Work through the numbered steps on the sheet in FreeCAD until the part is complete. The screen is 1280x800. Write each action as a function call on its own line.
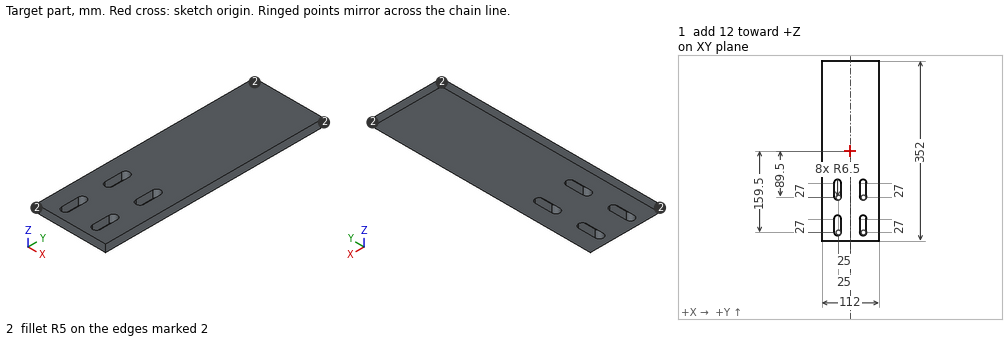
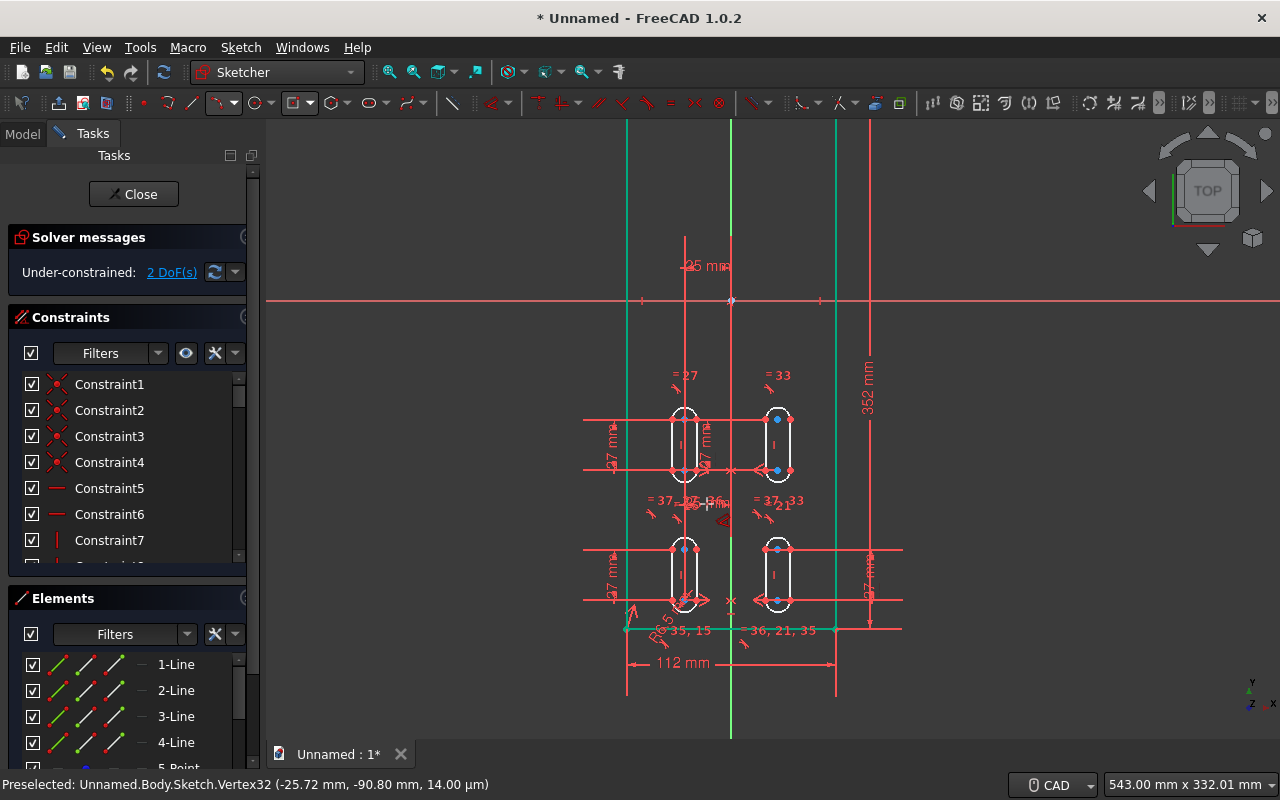
click(672, 470)
click(765, 385)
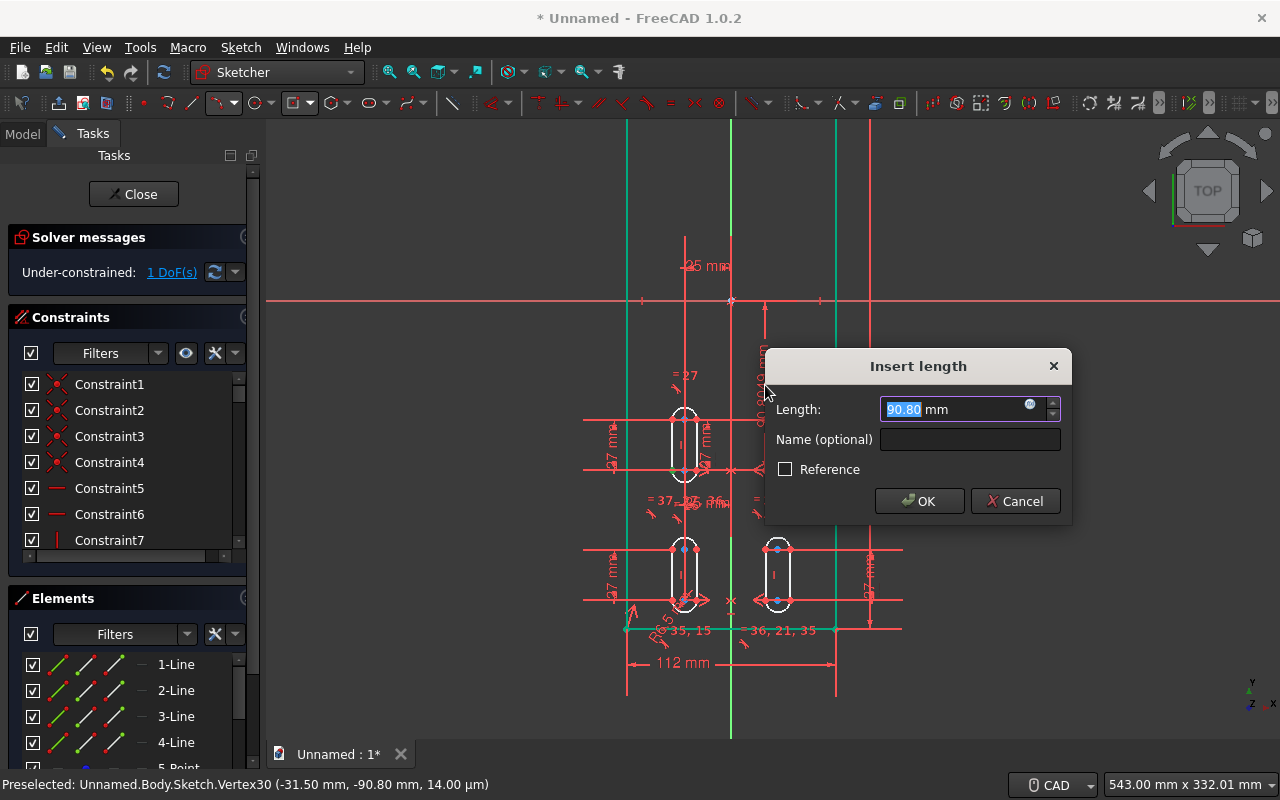
text(89.5)
key(Return)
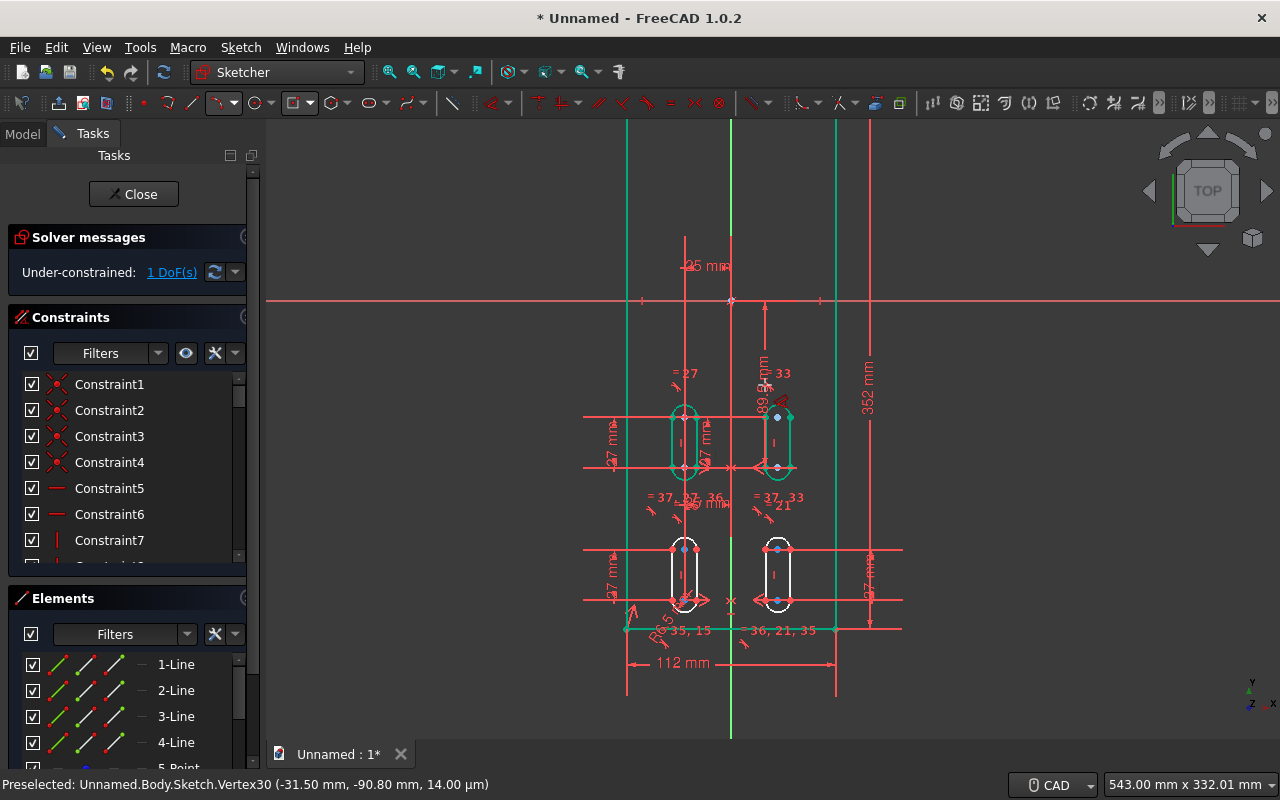
click(672, 600)
click(765, 346)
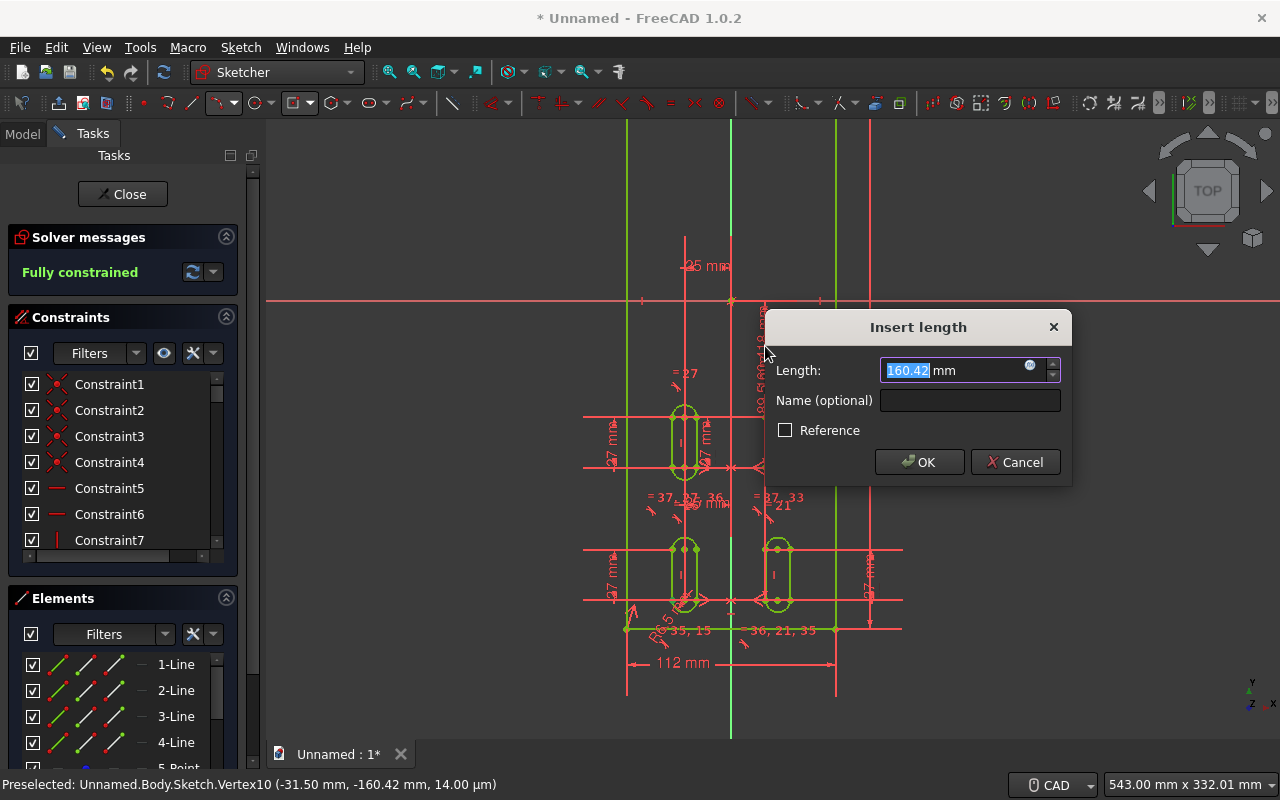
text(159.5)
key(Return)
key(Escape)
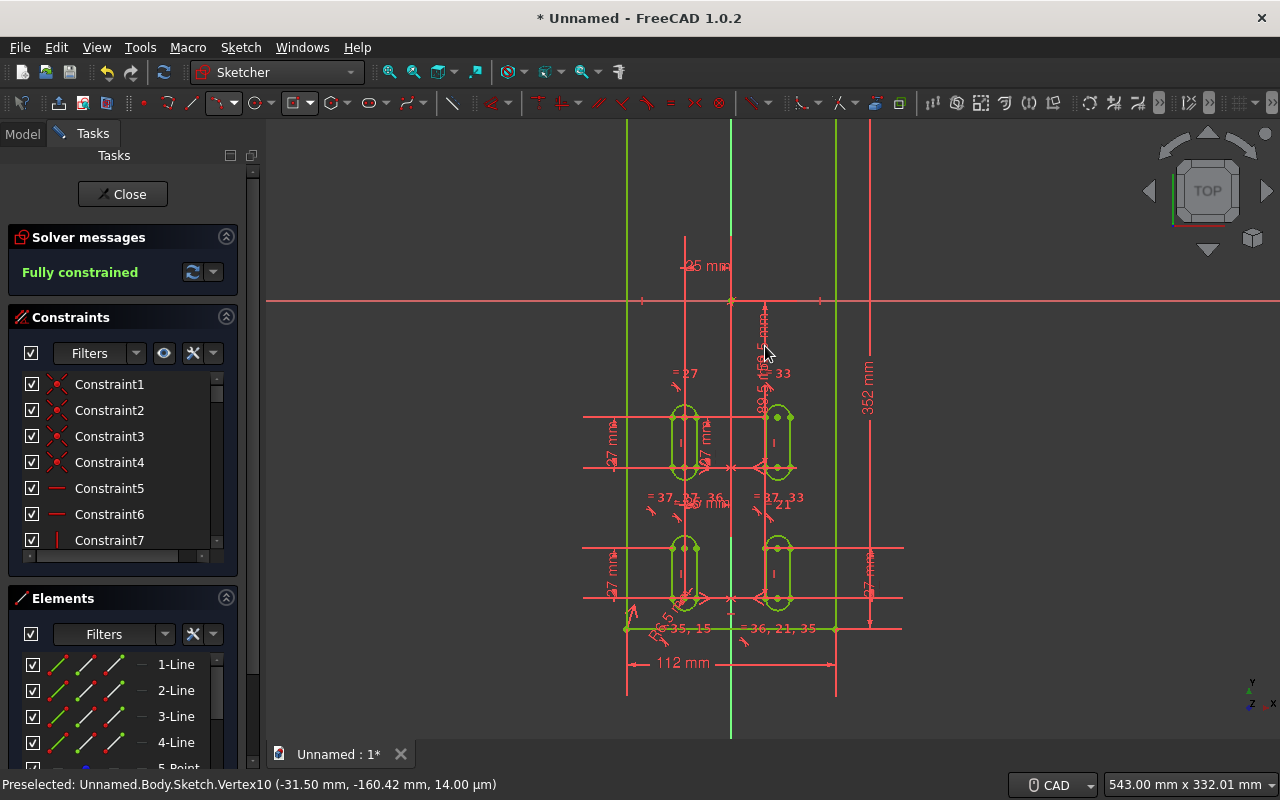
click(123, 194)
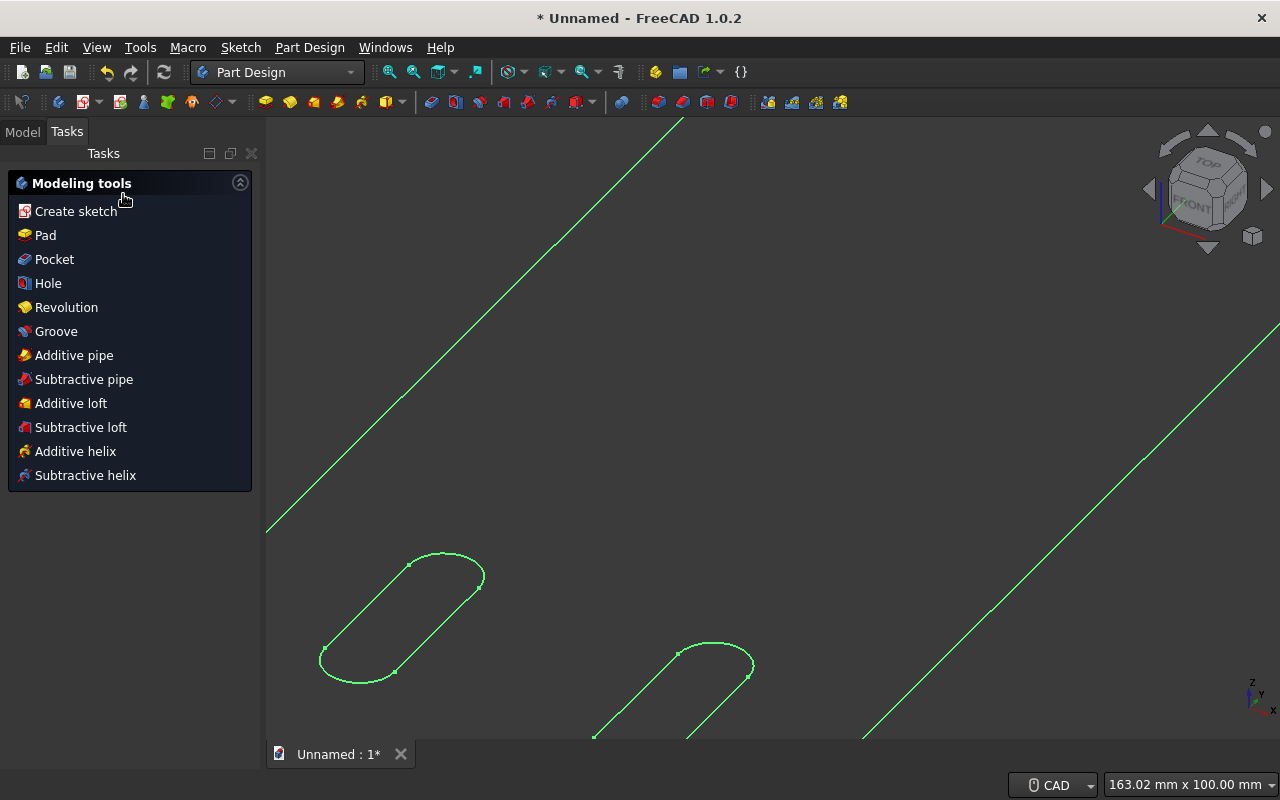
click(266, 102)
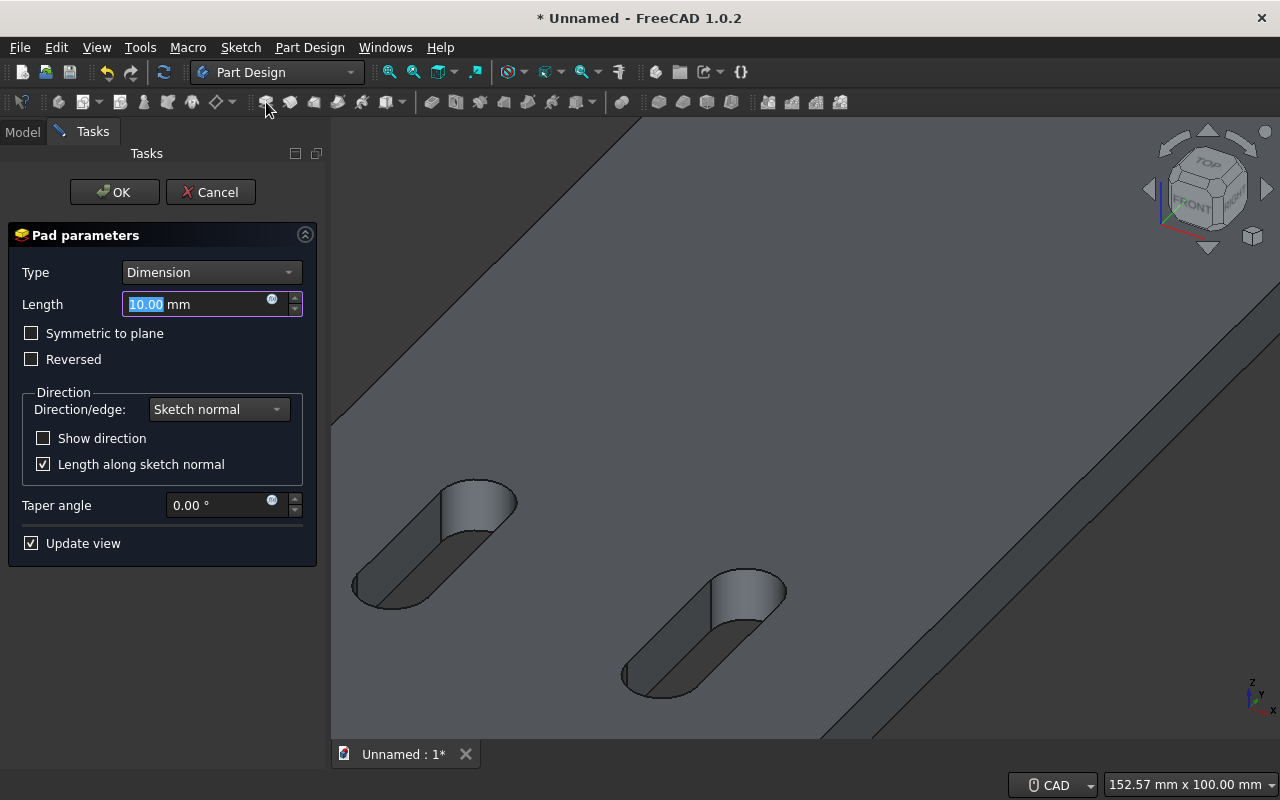
text(12)
key(Tab)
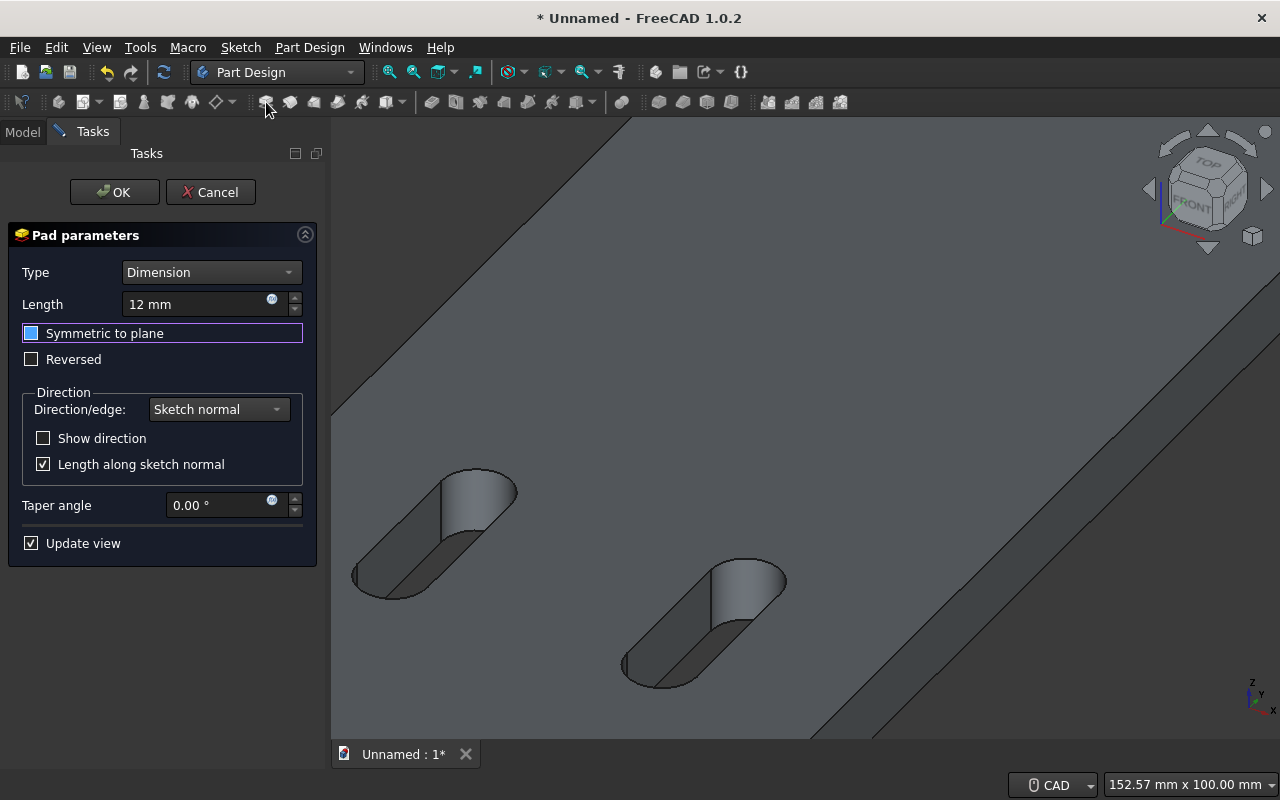
click(115, 192)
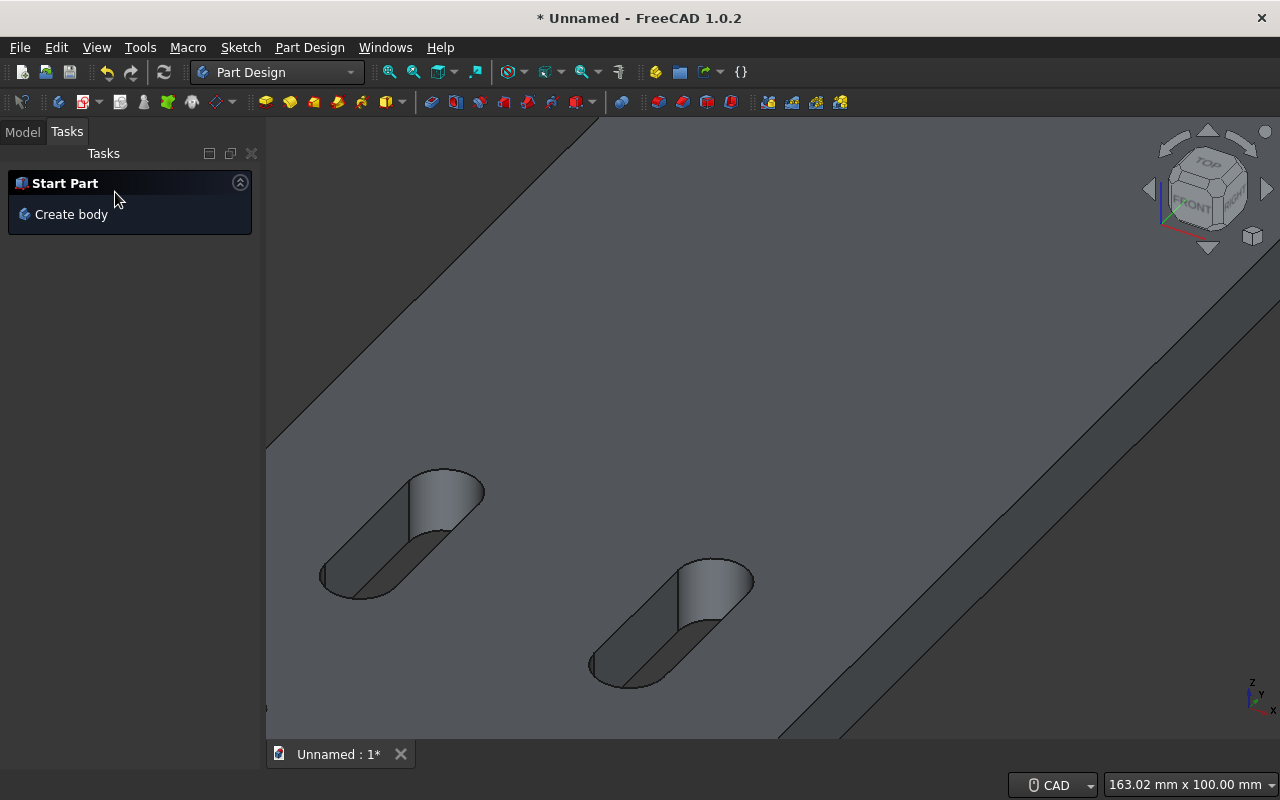
click(390, 72)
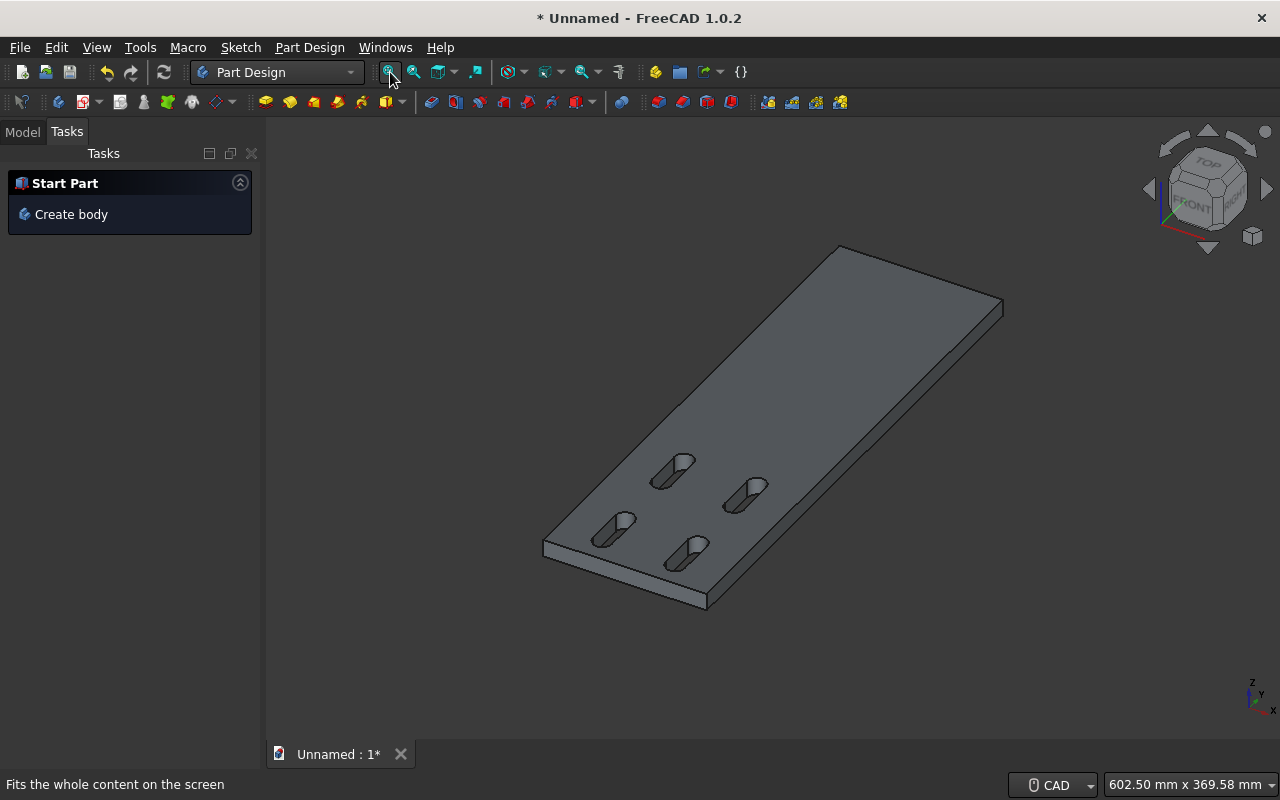
scroll(543, 547, up, 4)